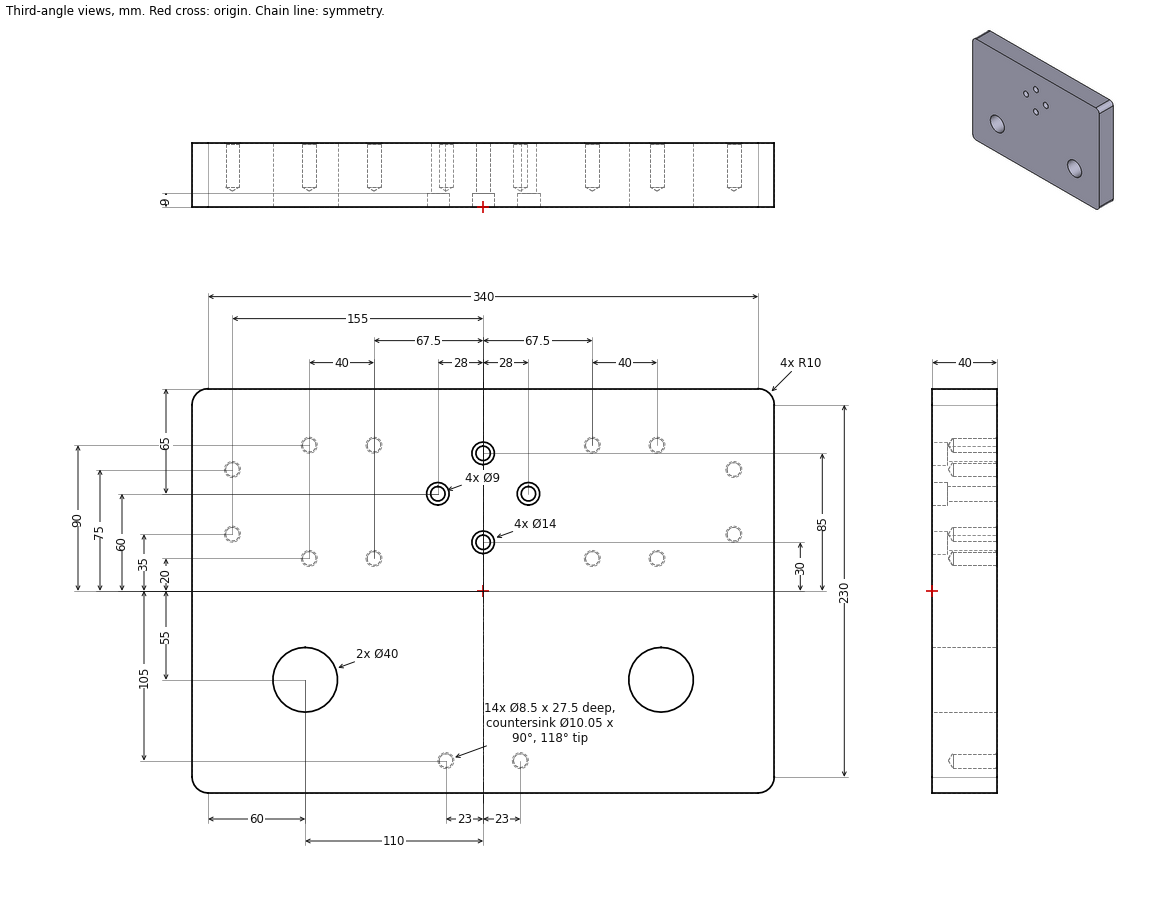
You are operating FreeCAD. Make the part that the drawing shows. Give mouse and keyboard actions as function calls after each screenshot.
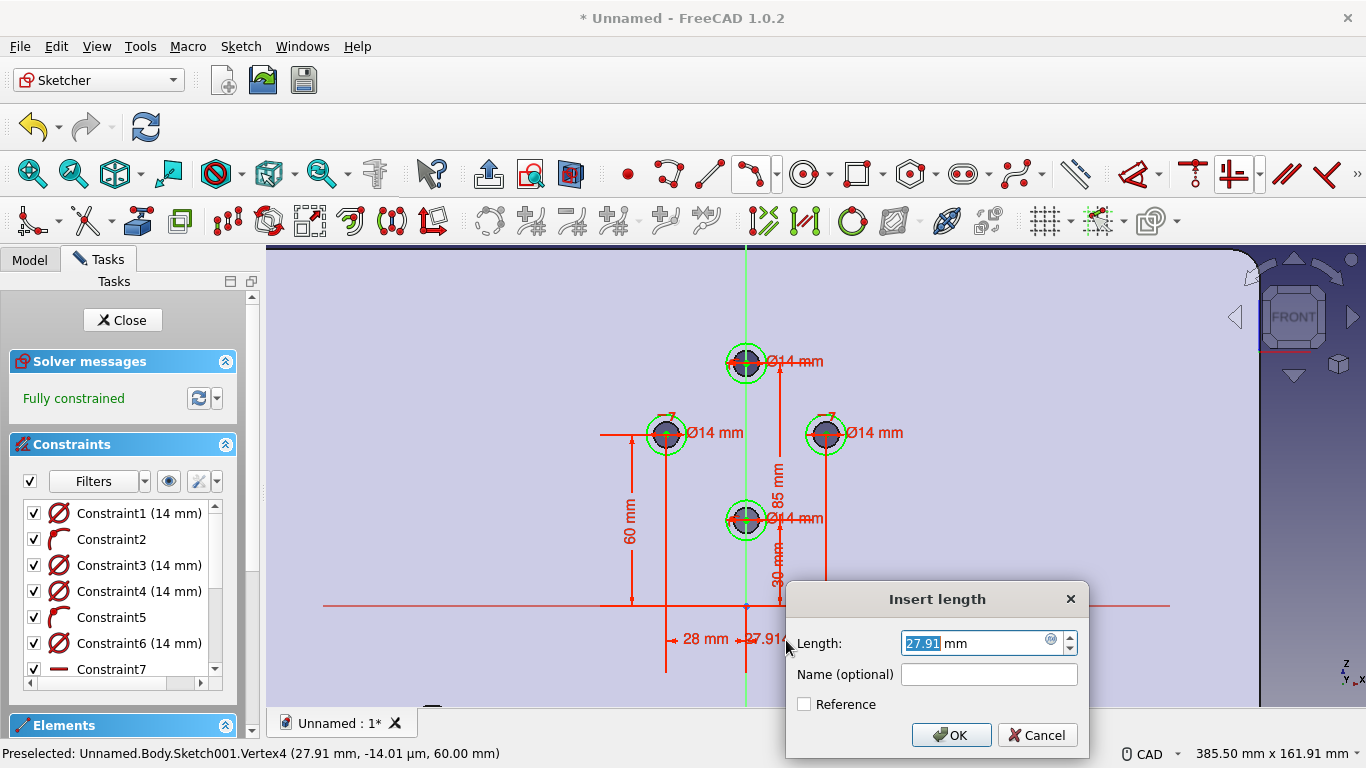
text(28)
key(Return)
key(Escape)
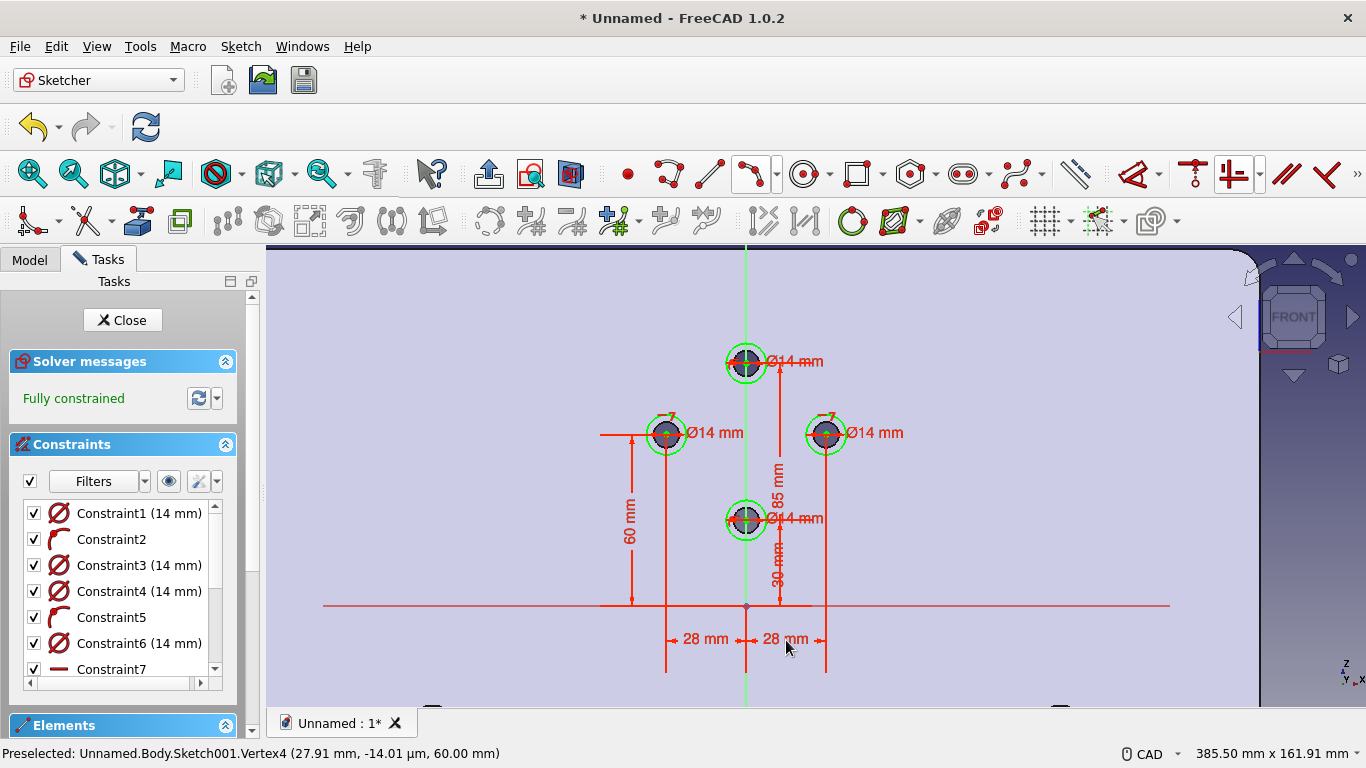
click(123, 320)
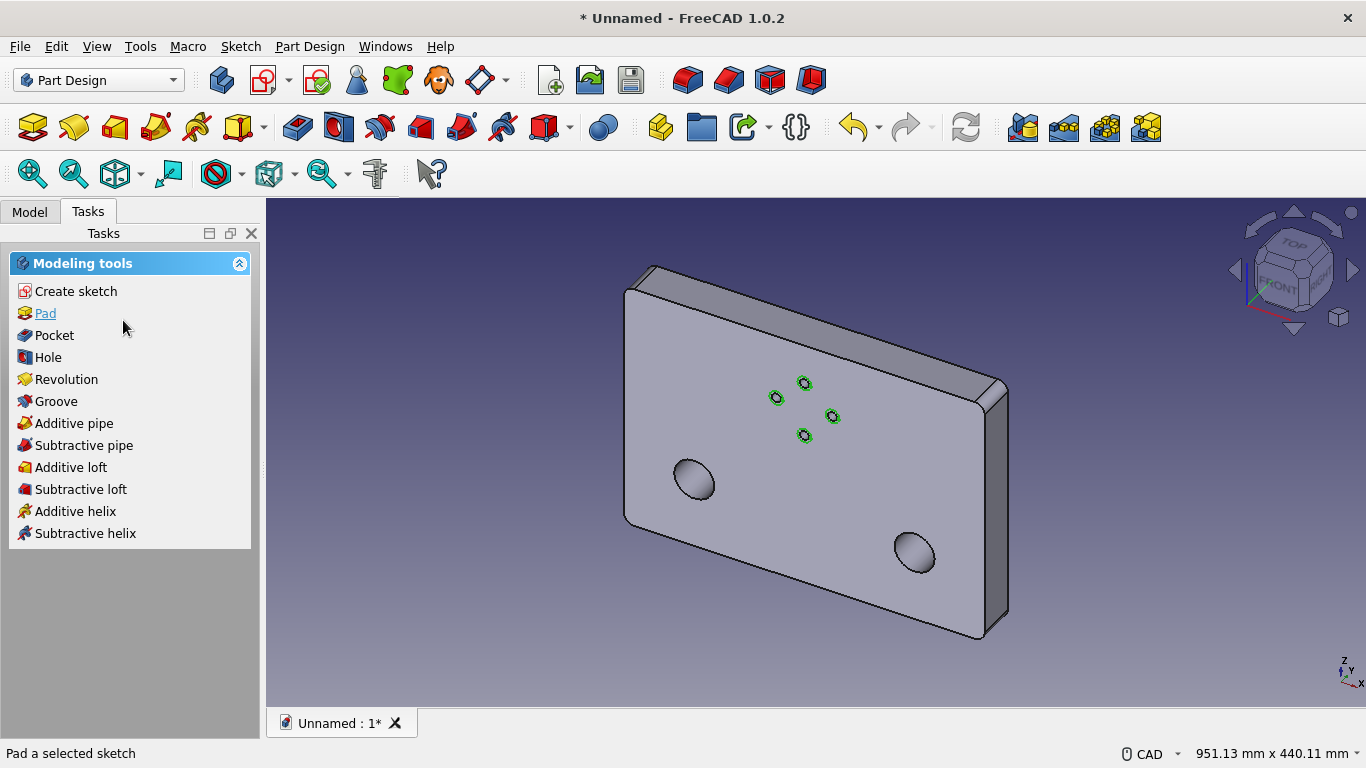
click(298, 128)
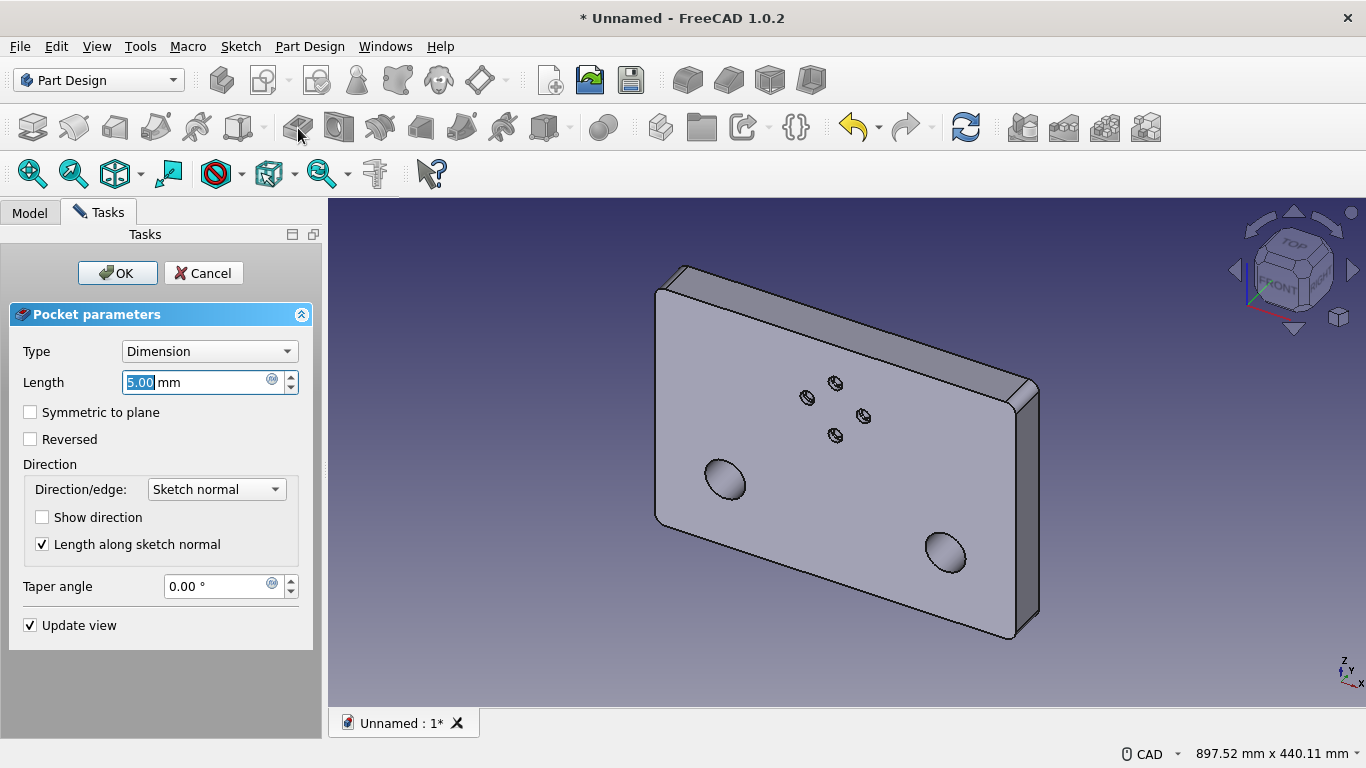
text(9)
key(Tab)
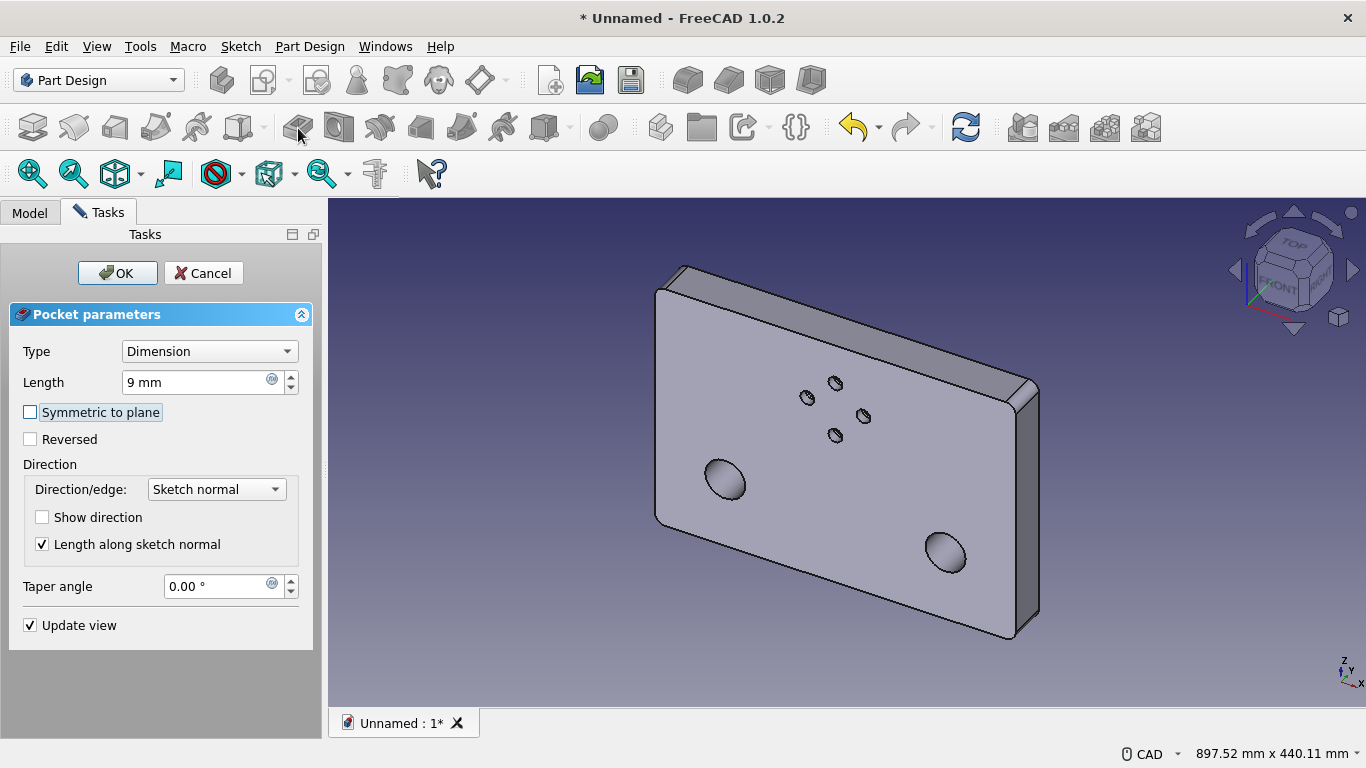
click(118, 273)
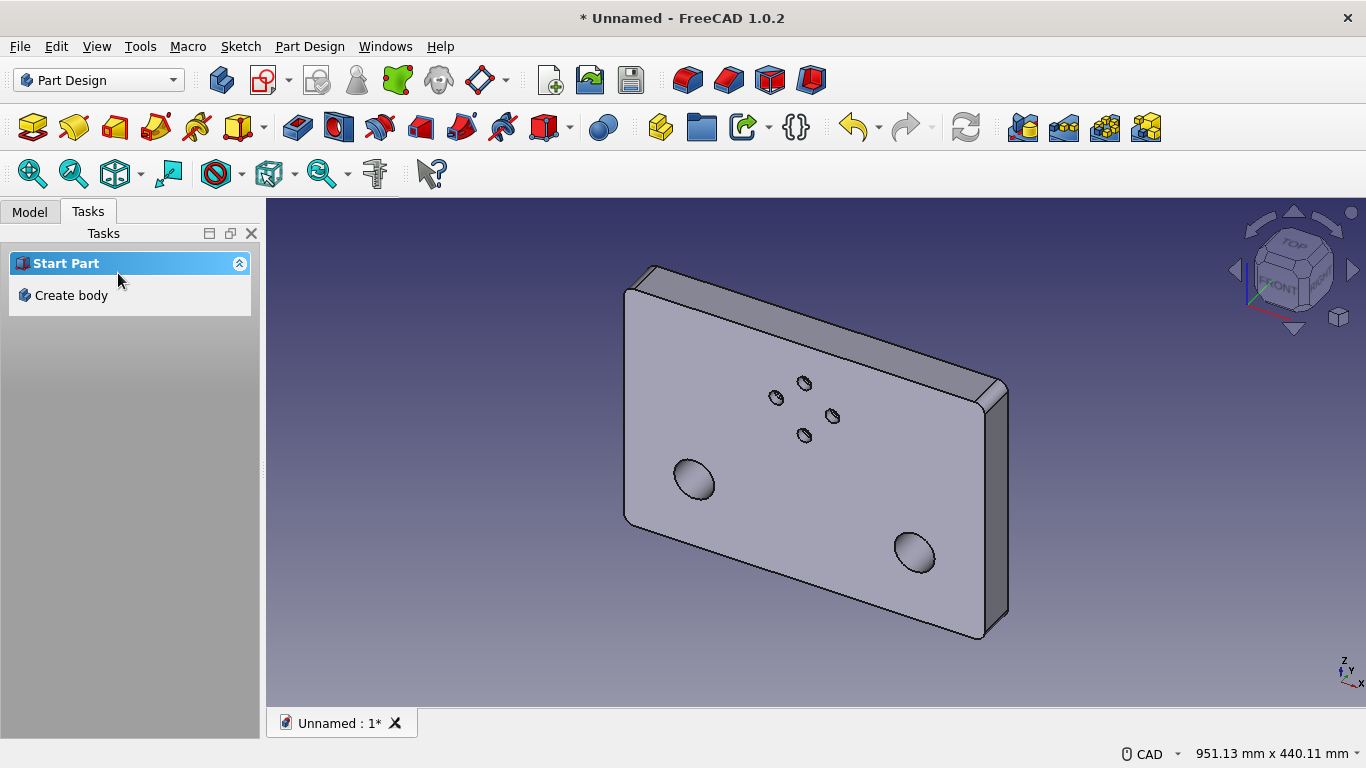
key(4)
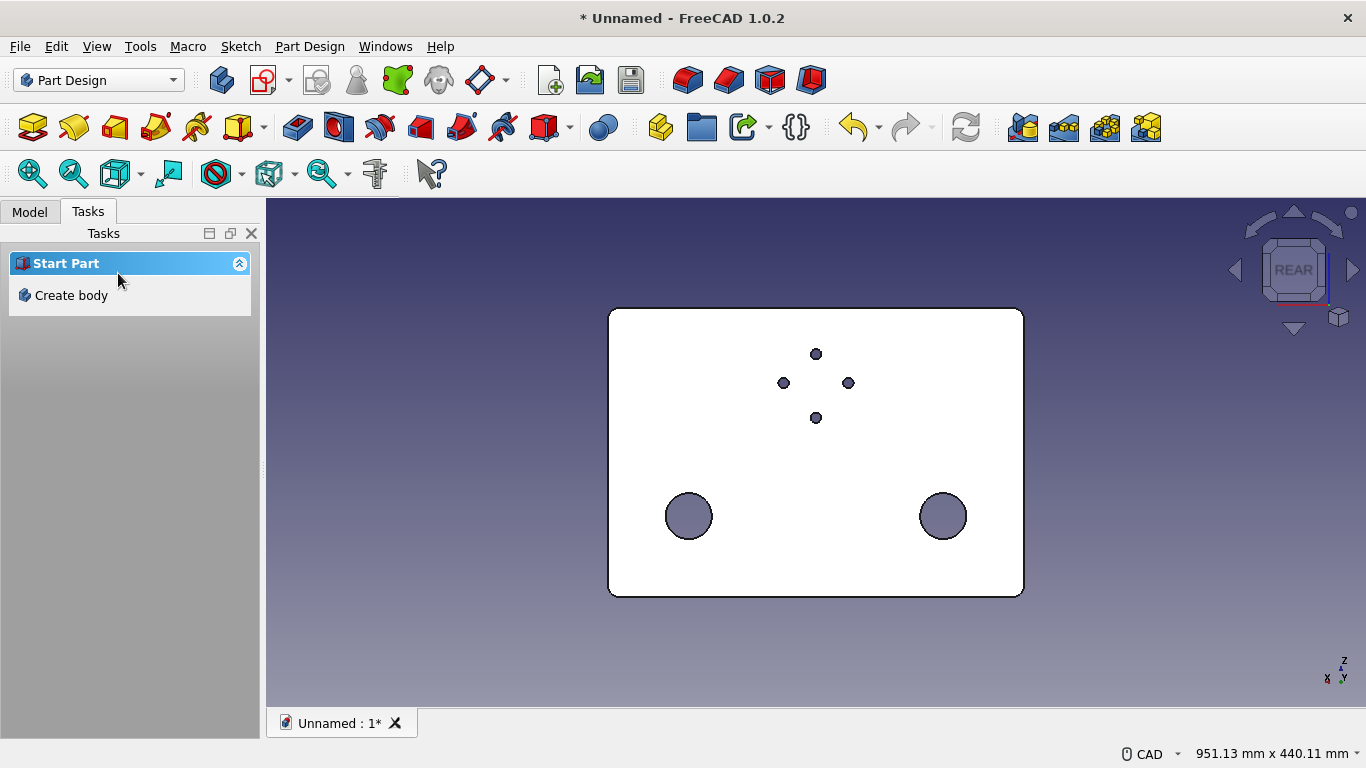
click(935, 410)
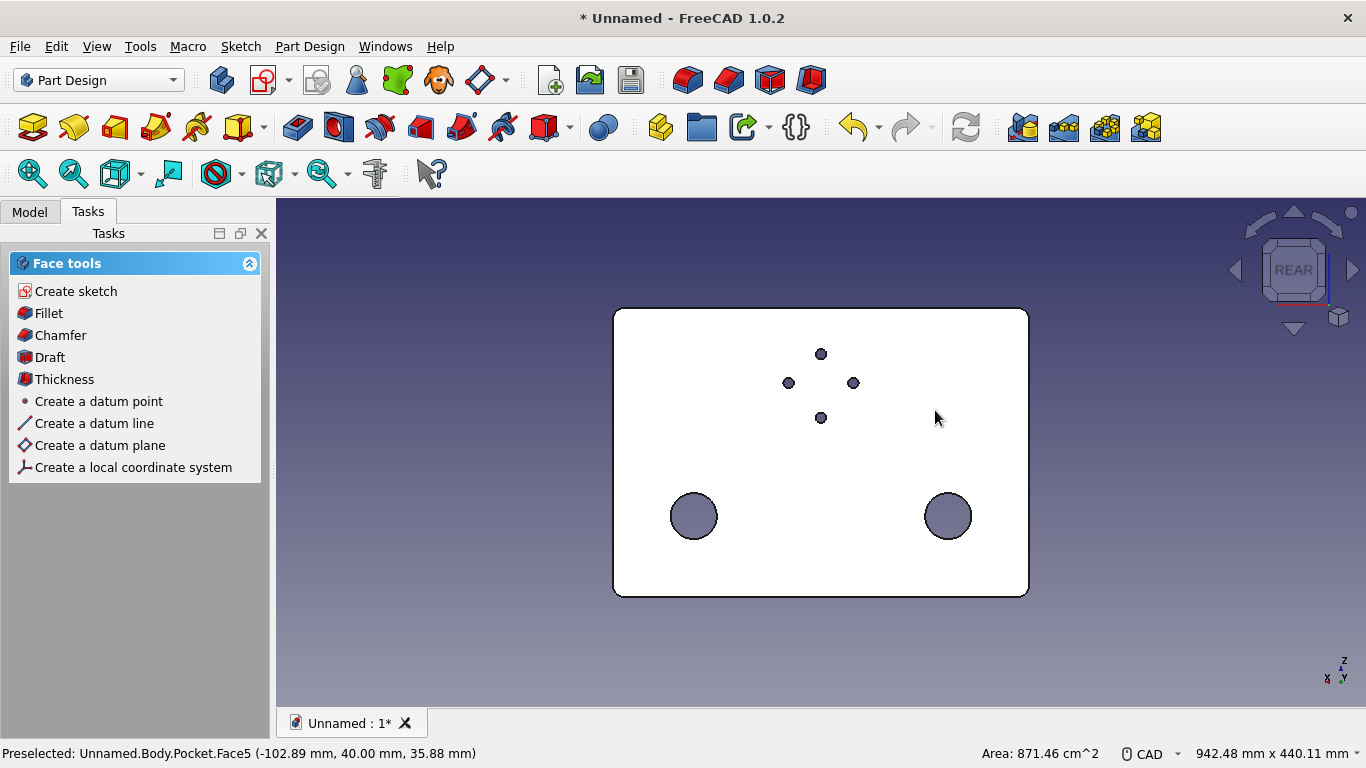
click(262, 80)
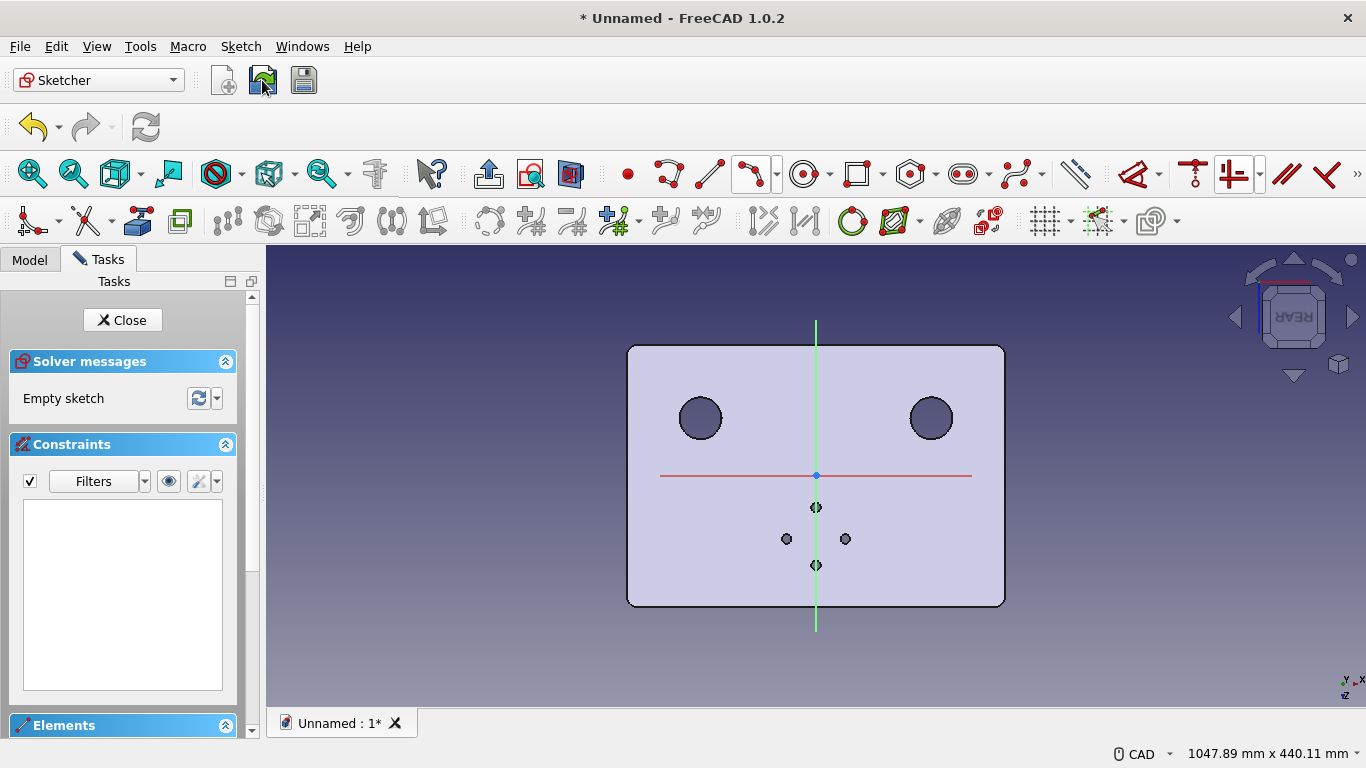
click(804, 174)